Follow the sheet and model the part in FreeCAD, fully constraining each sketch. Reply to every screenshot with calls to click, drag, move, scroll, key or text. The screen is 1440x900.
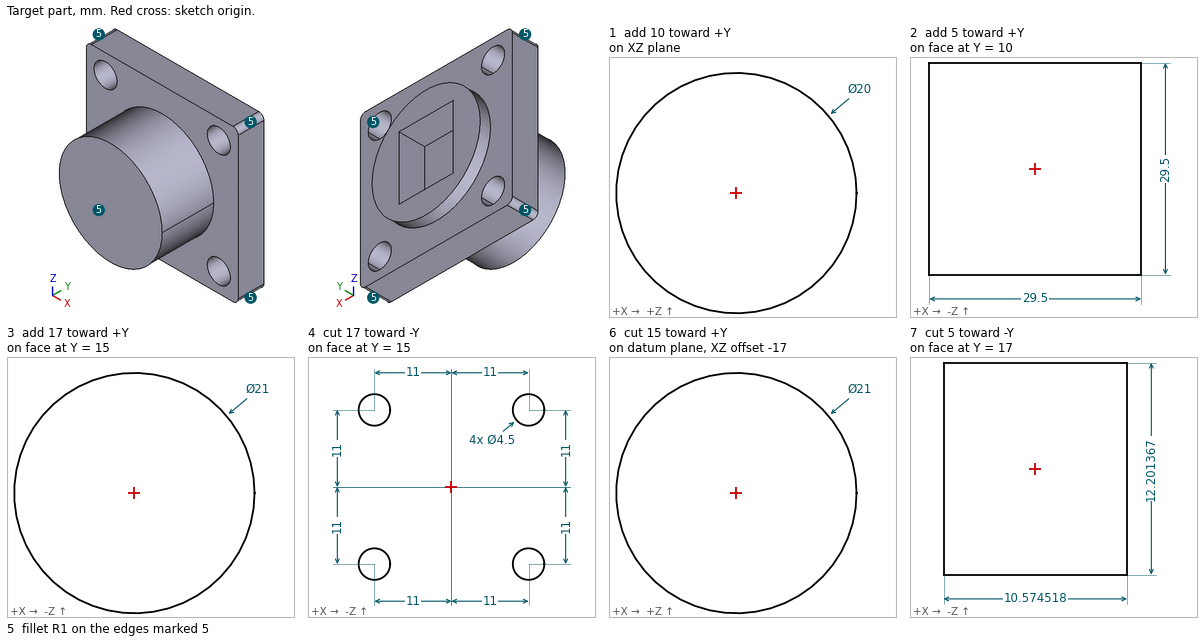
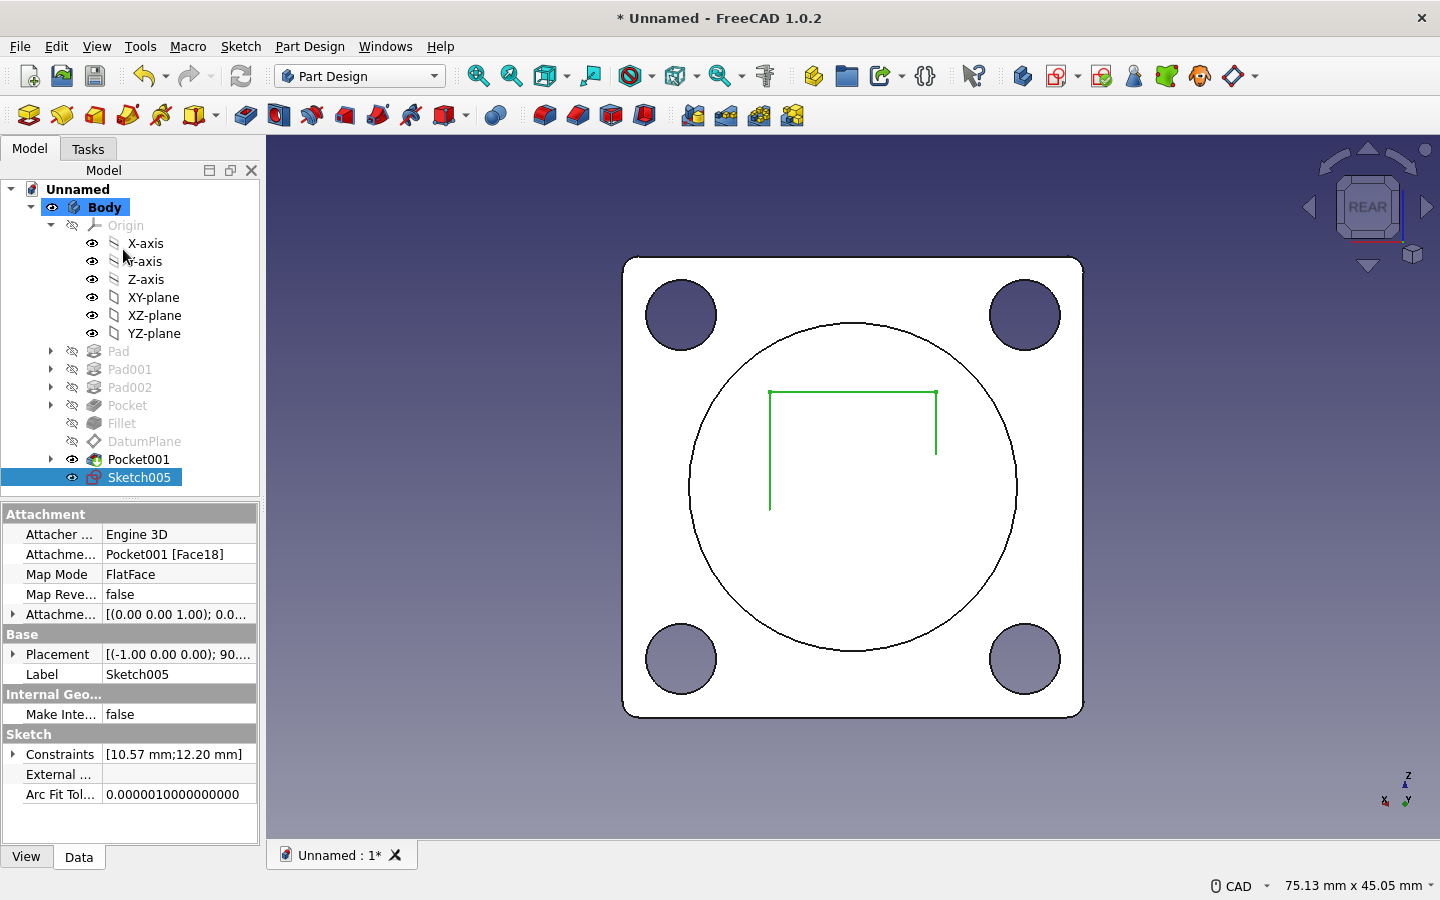
click(246, 116)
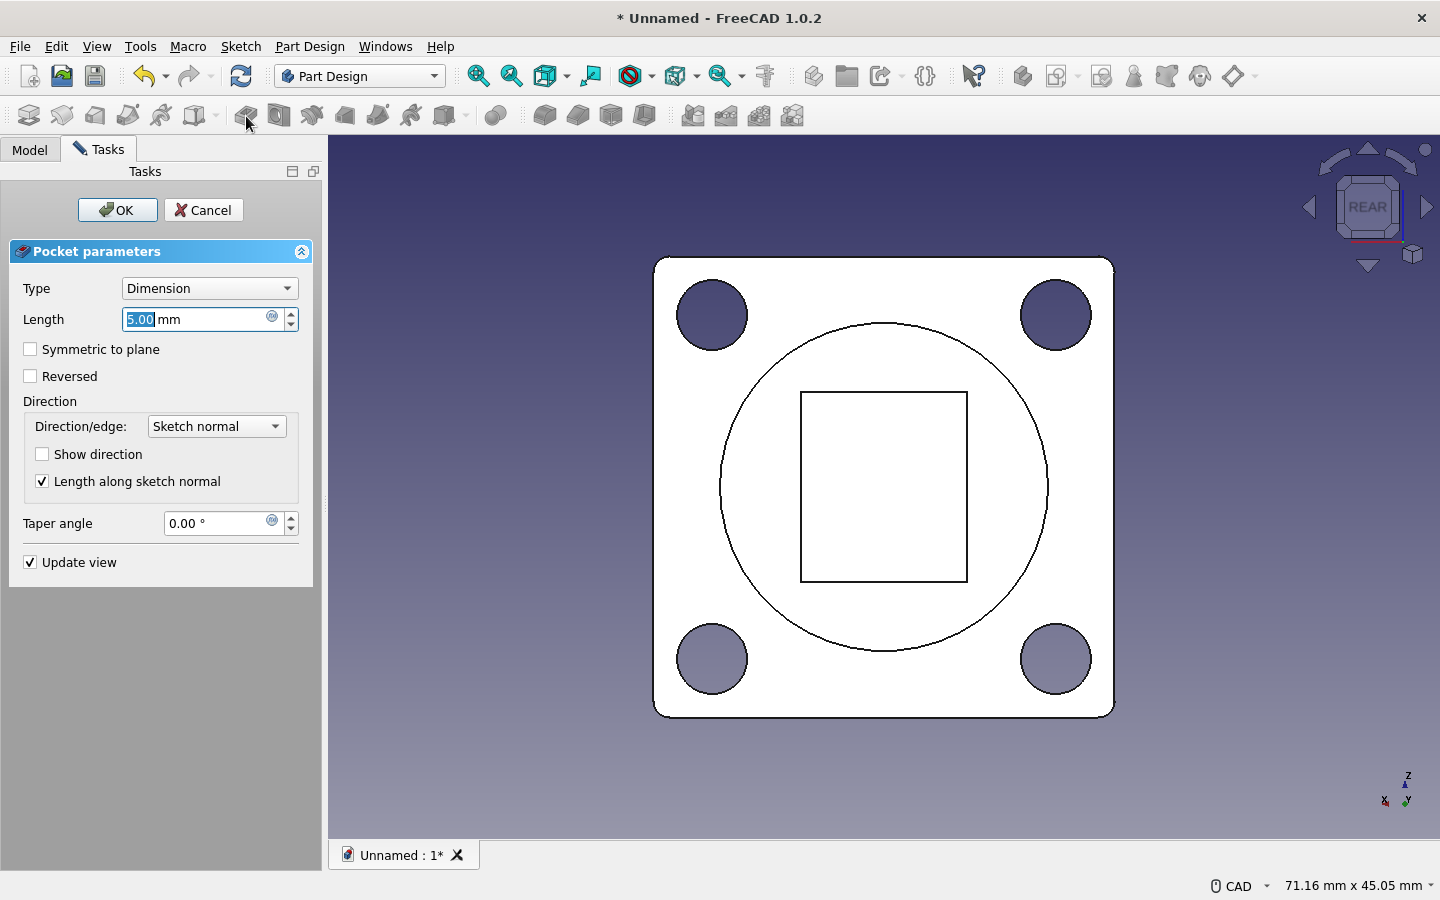
text(5)
key(Tab)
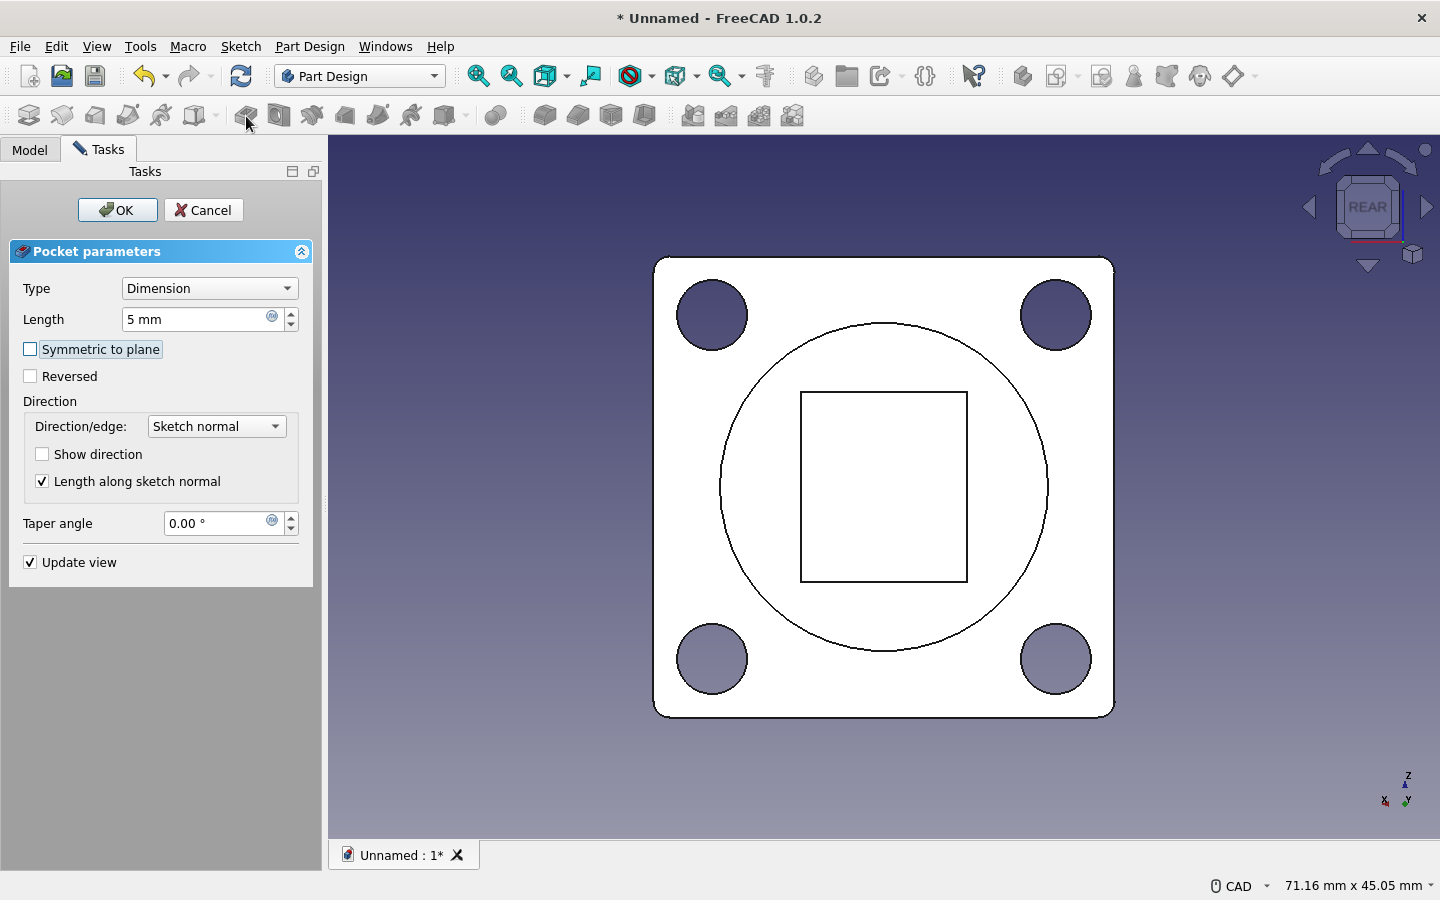
click(118, 210)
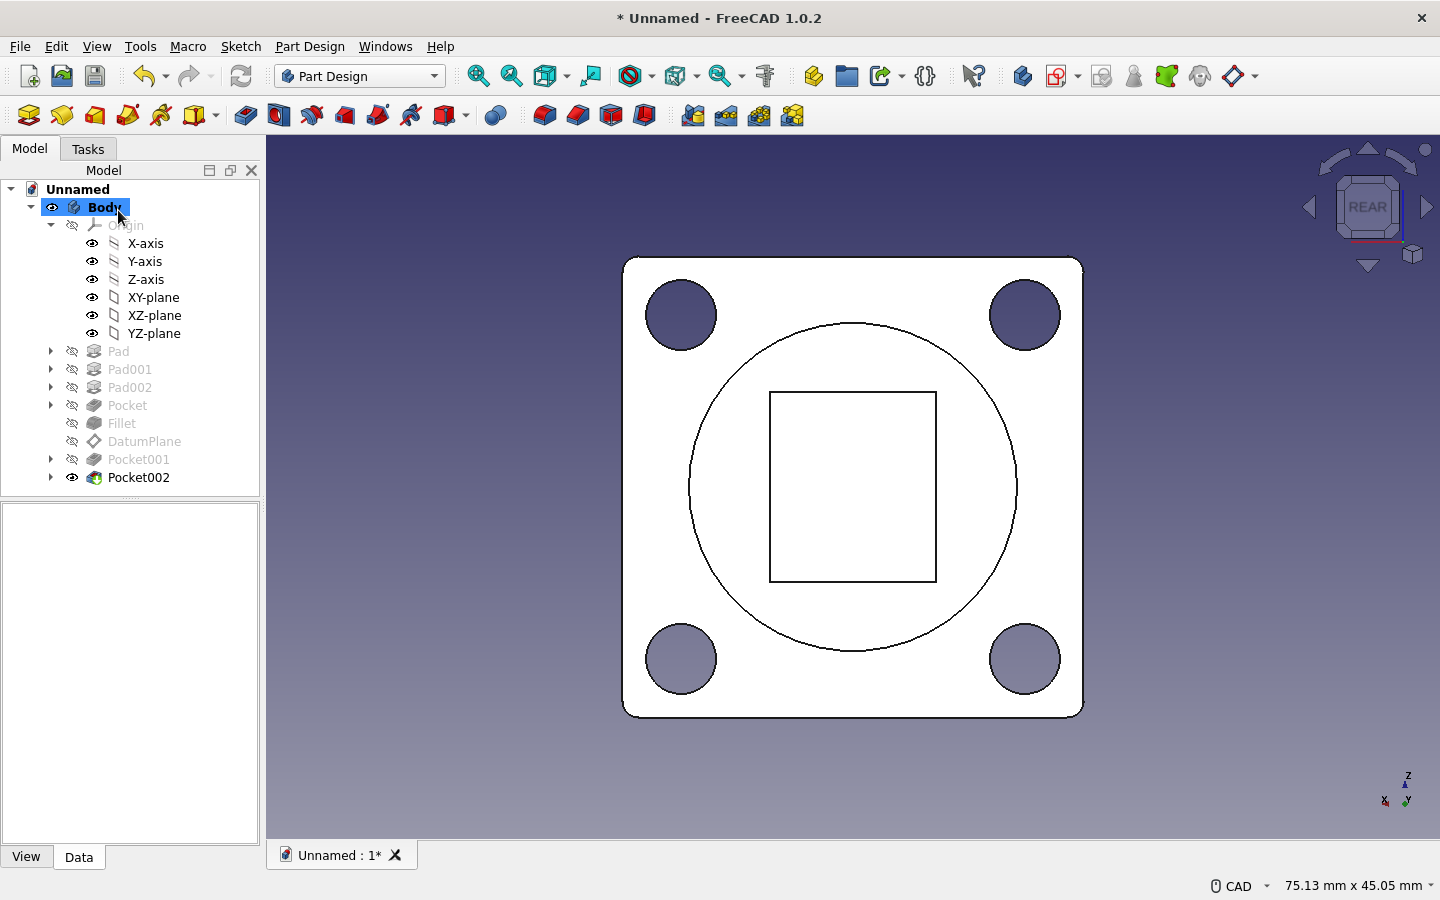
key(0)